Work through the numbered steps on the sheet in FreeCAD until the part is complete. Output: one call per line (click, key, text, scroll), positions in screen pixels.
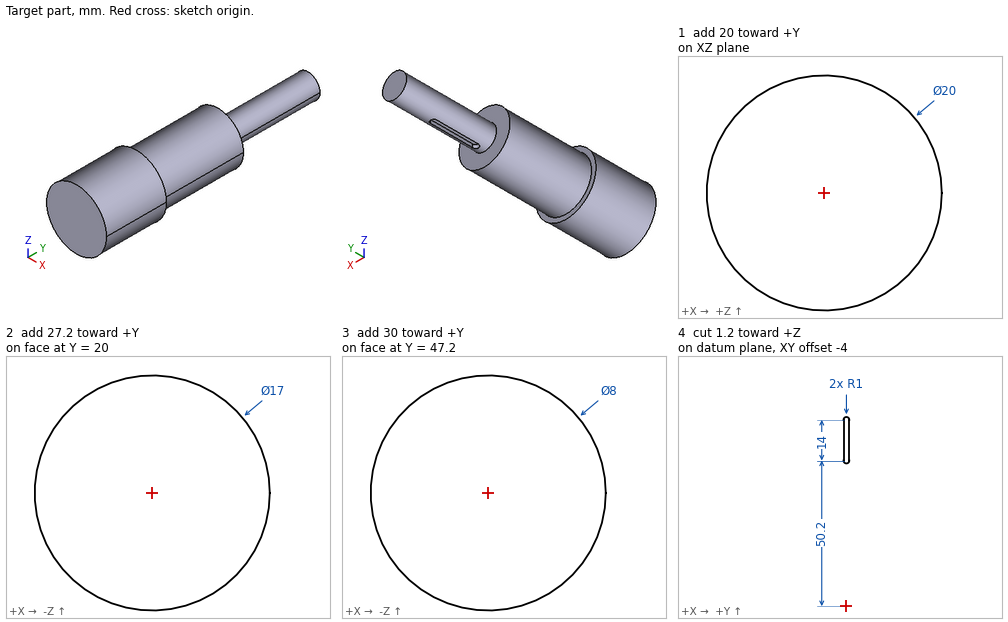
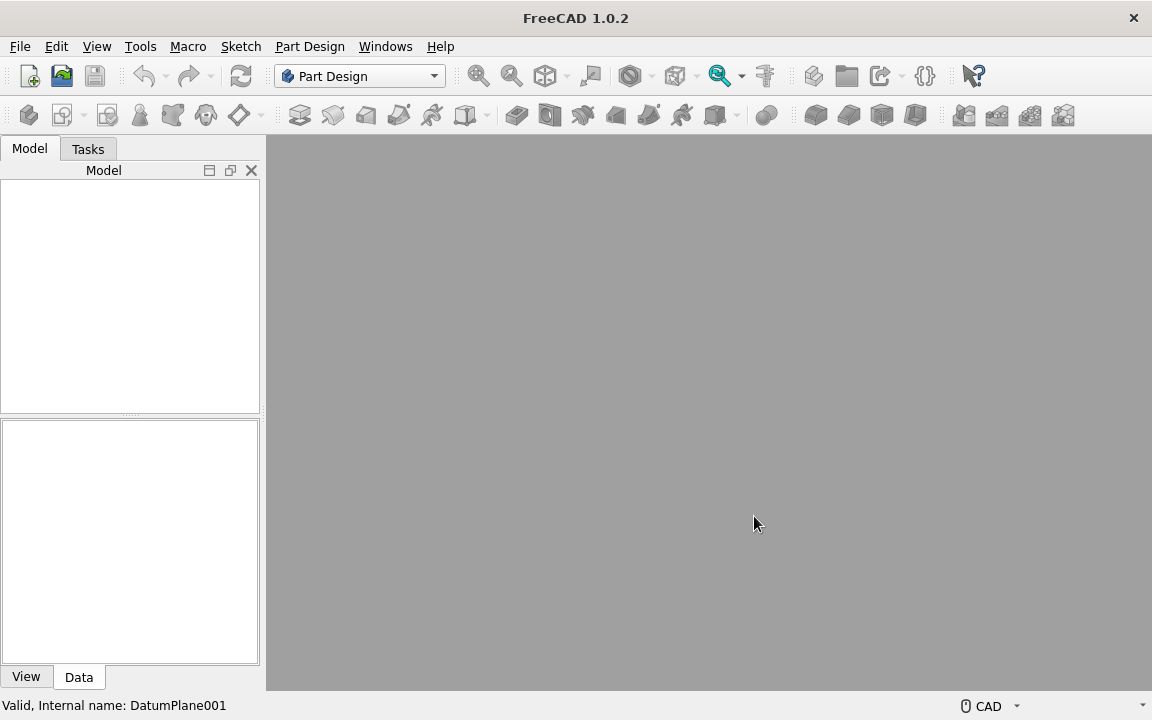
click(29, 76)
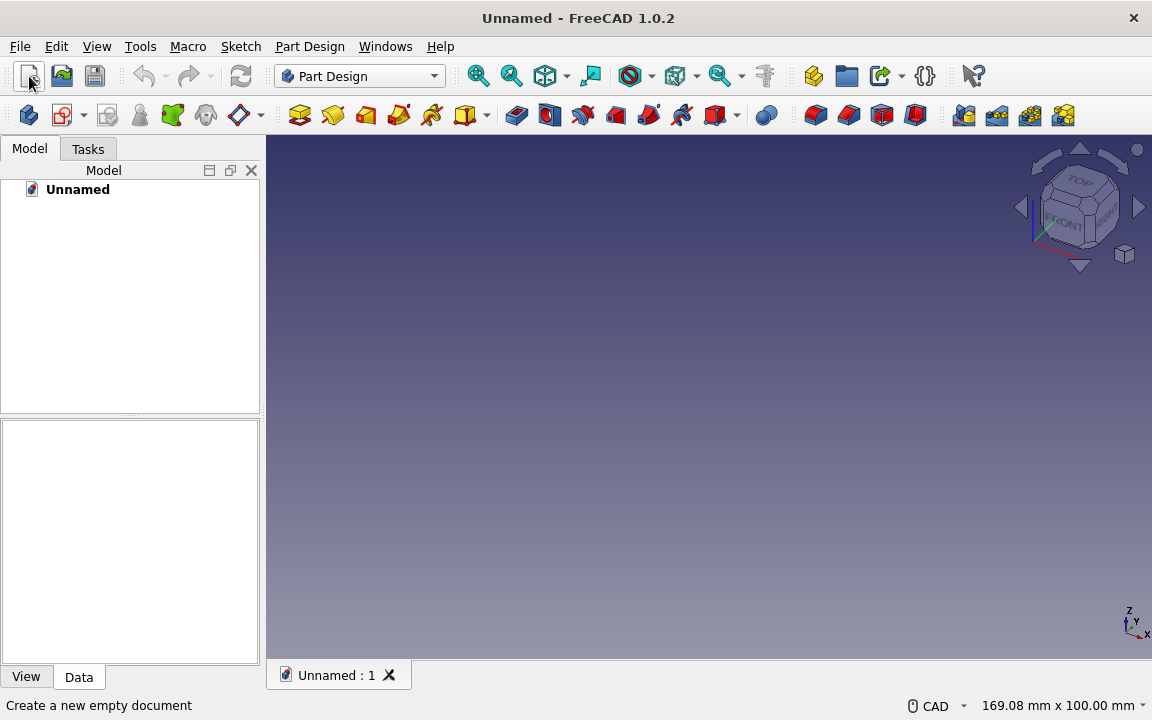
click(62, 116)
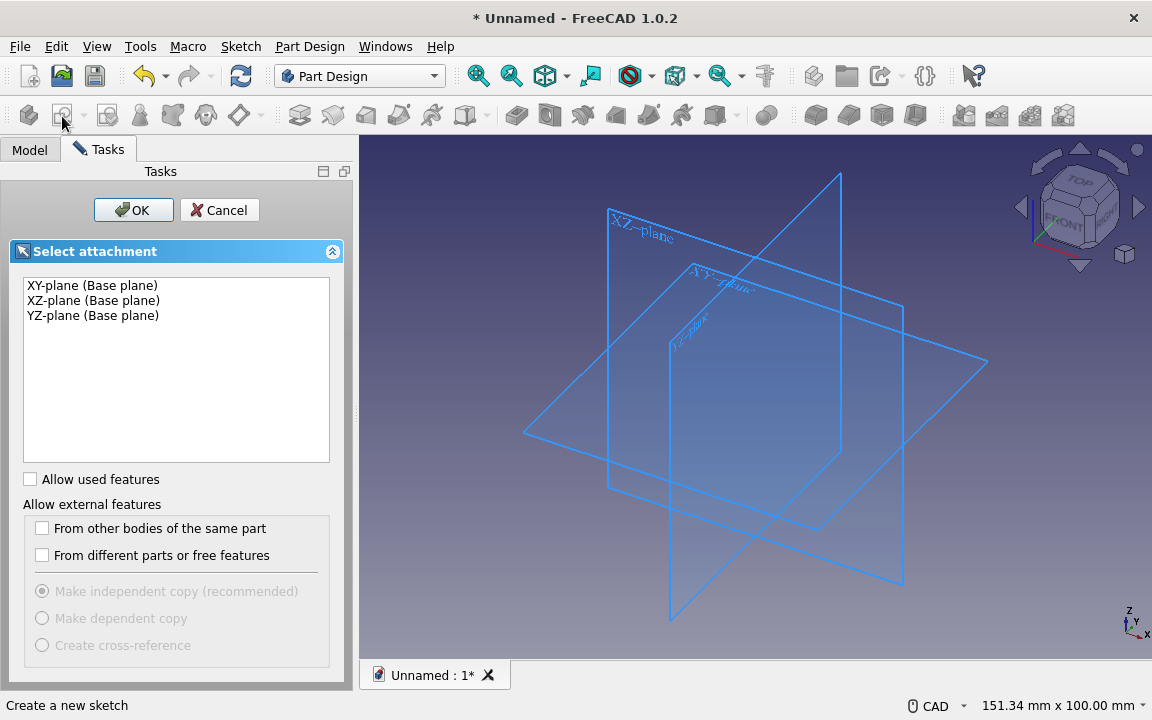
click(84, 300)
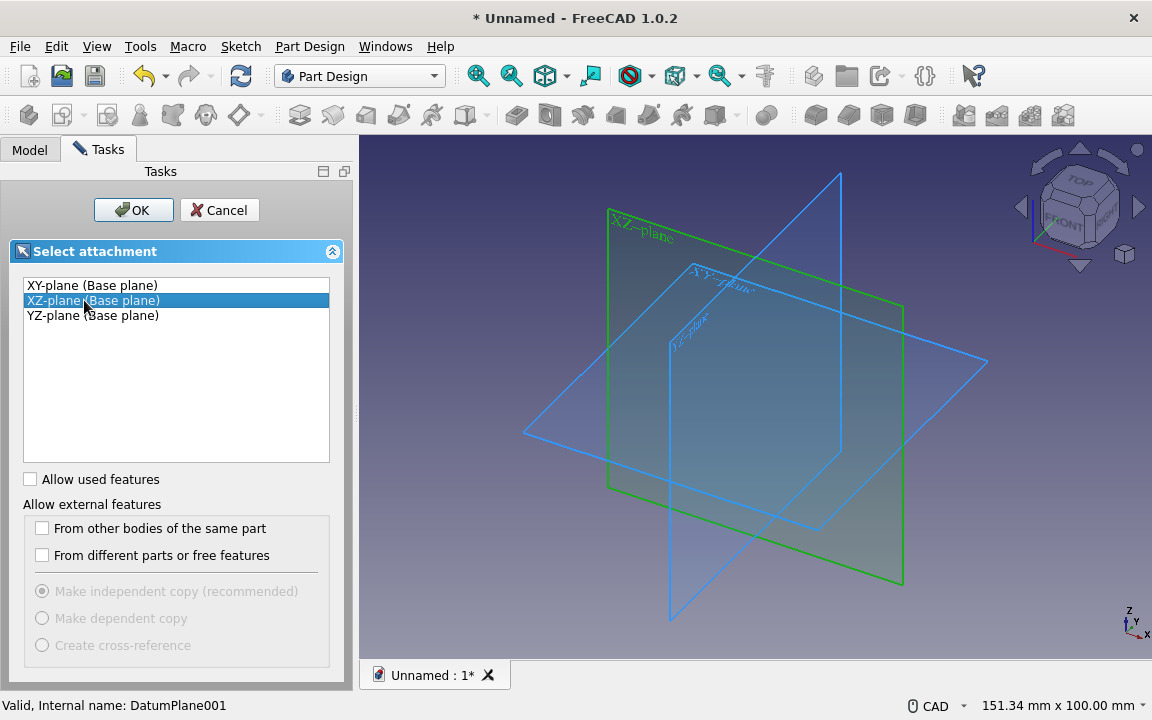
click(134, 210)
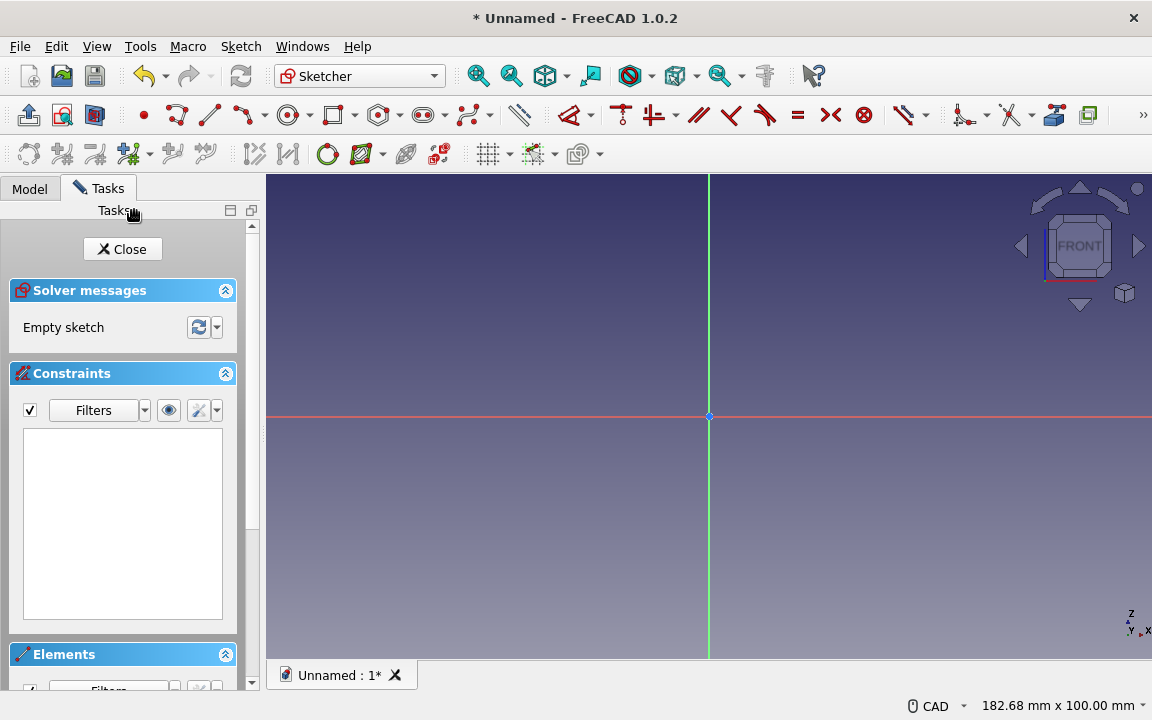
scroll(739, 416, up, 6)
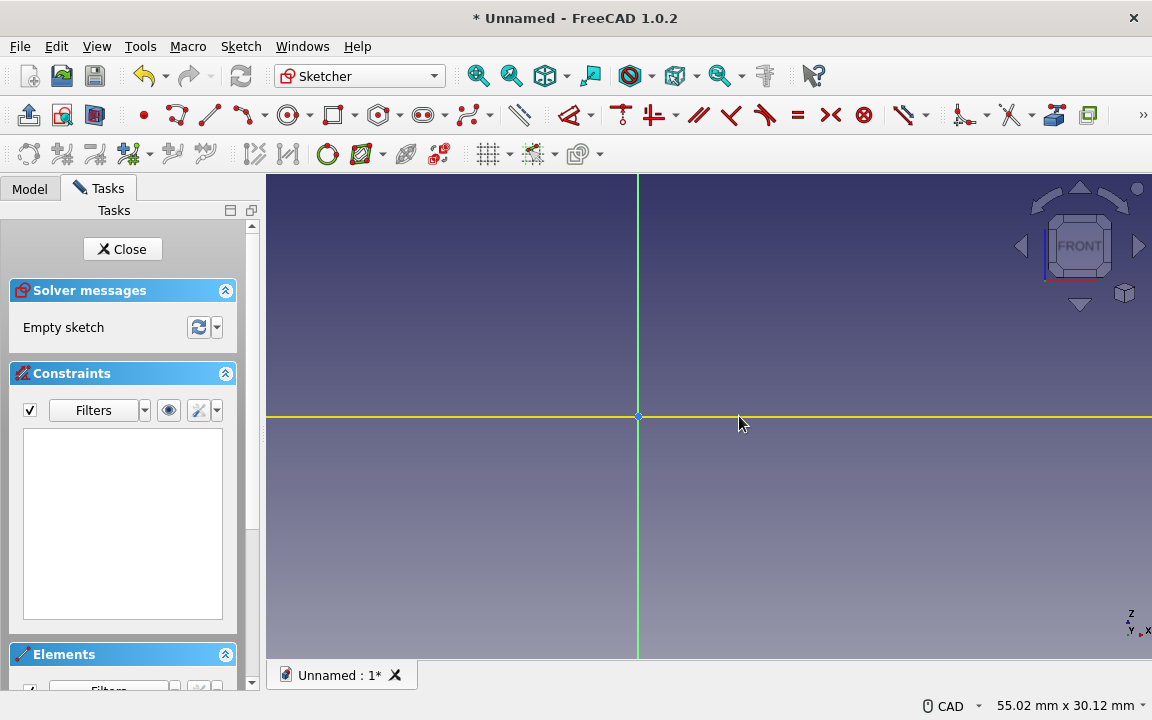
click(288, 116)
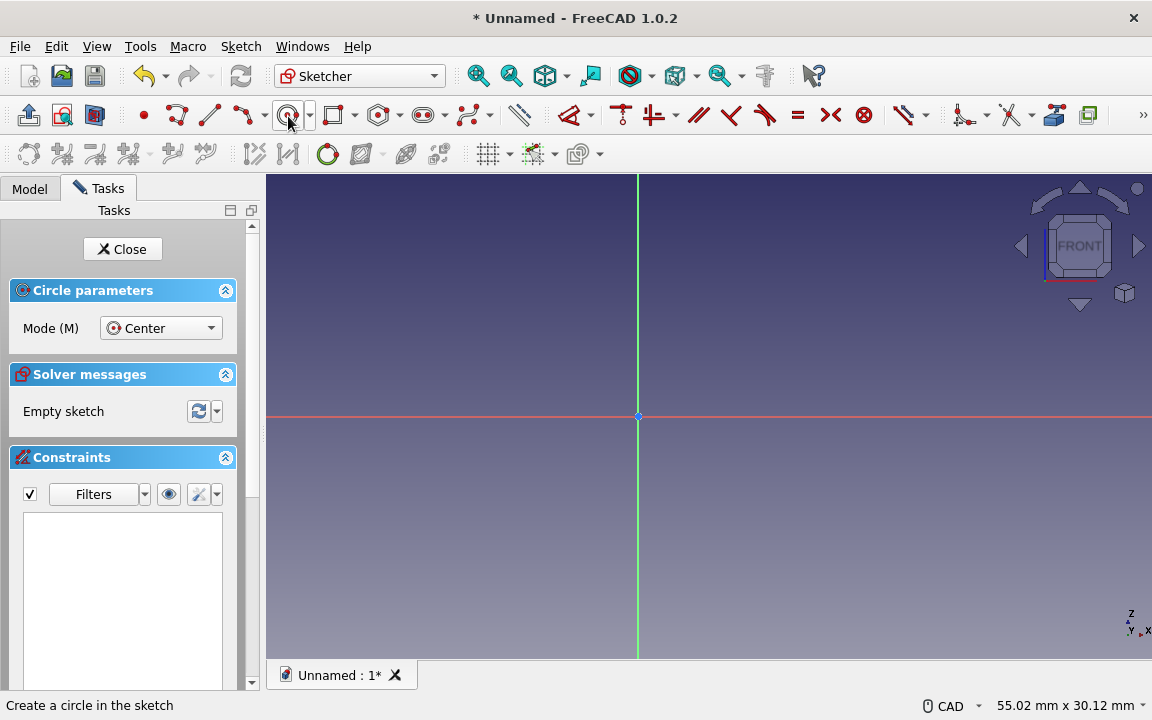
click(638, 416)
move(752, 303)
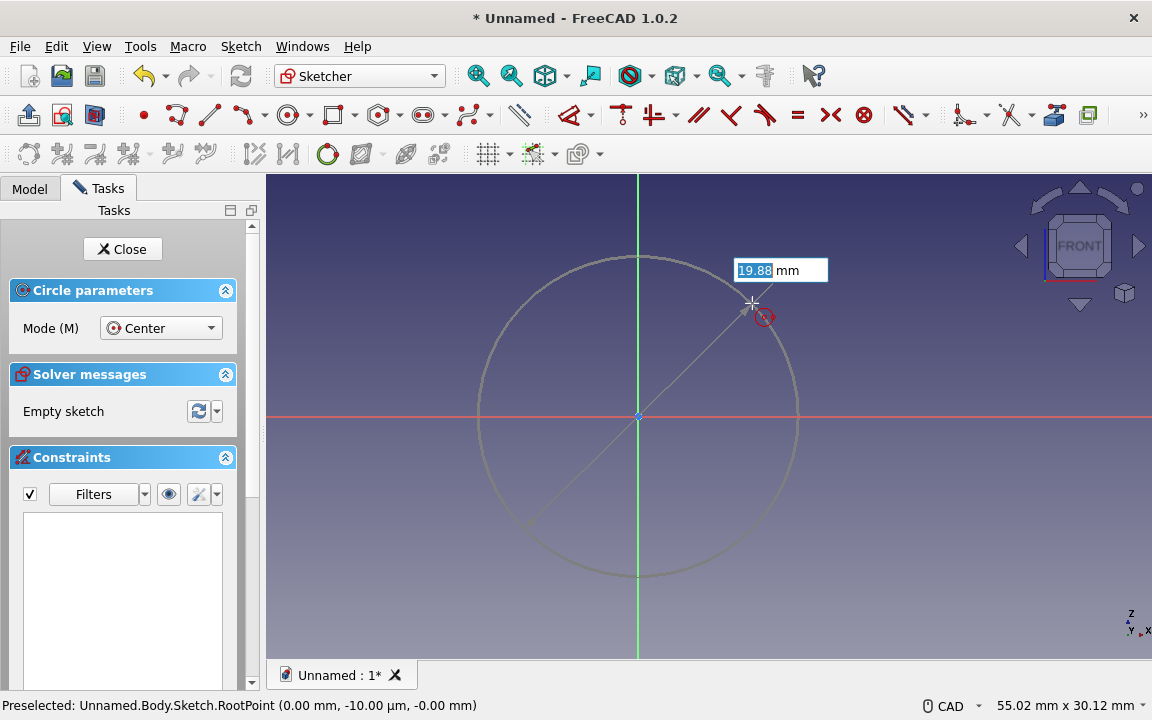
text(20)
key(Return)
key(Escape)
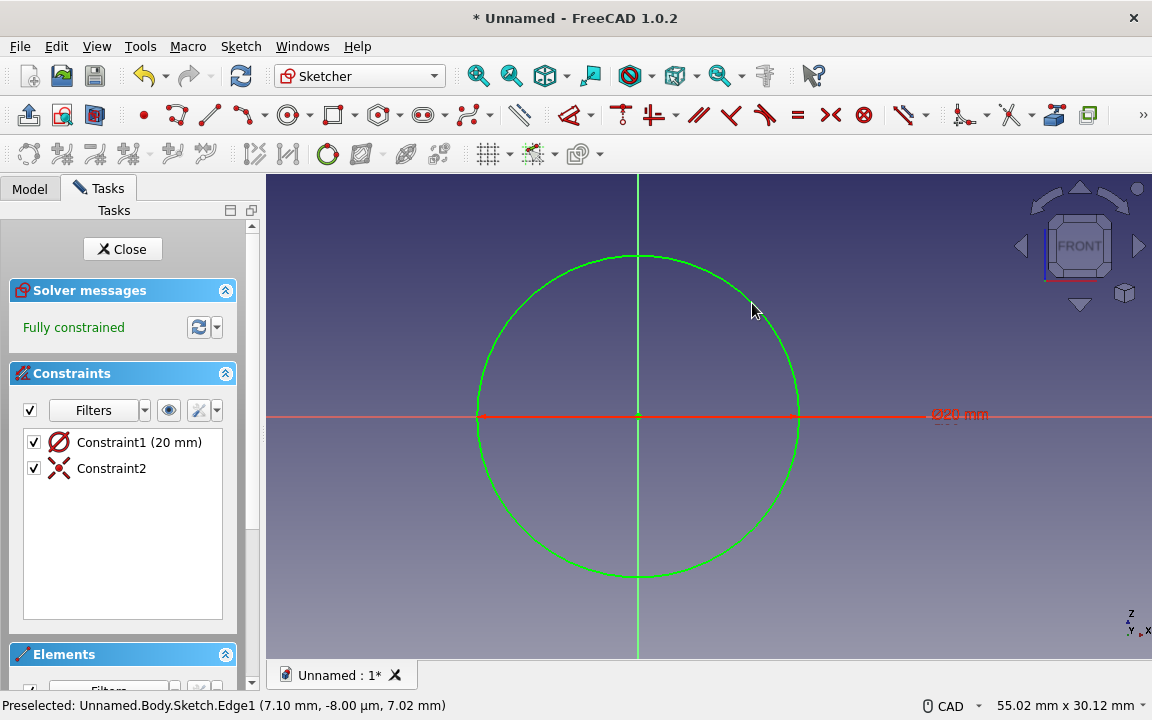
click(123, 249)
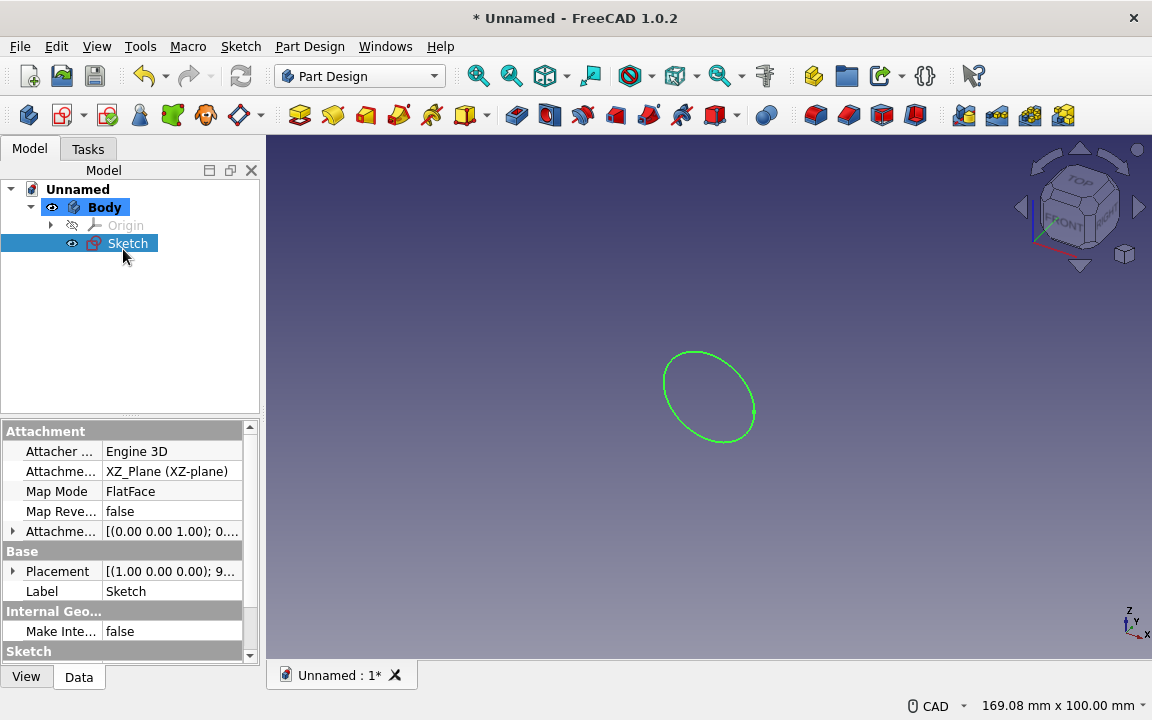
click(300, 116)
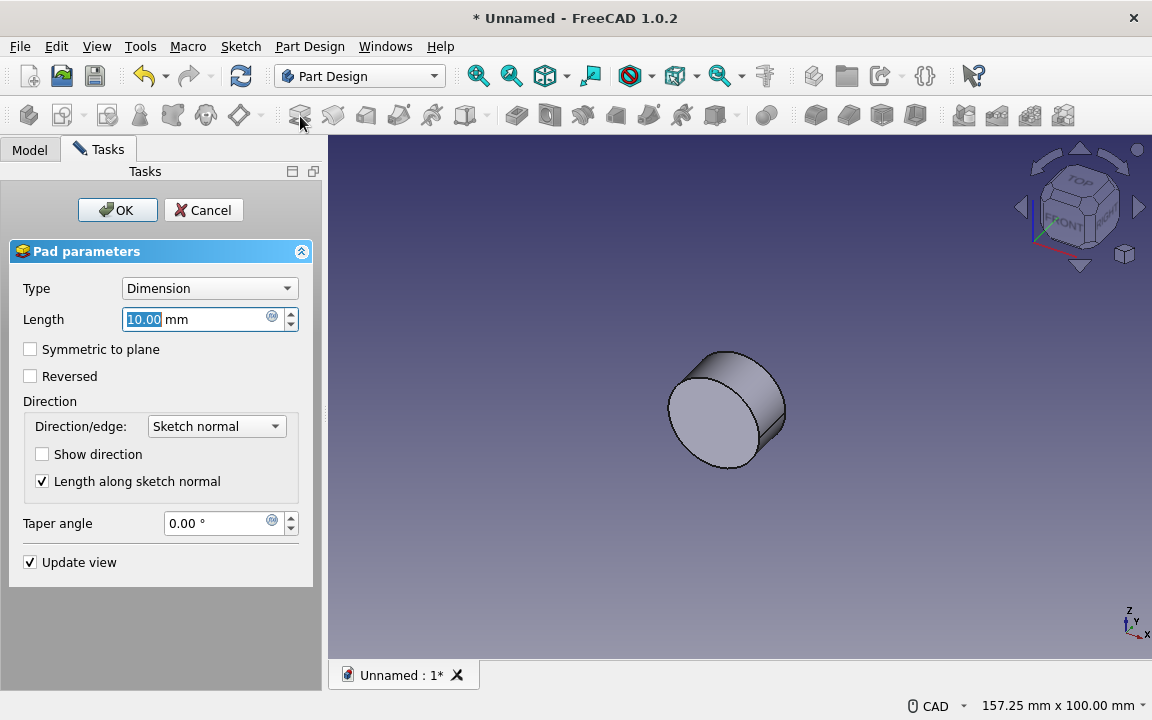
text(20)
key(Tab)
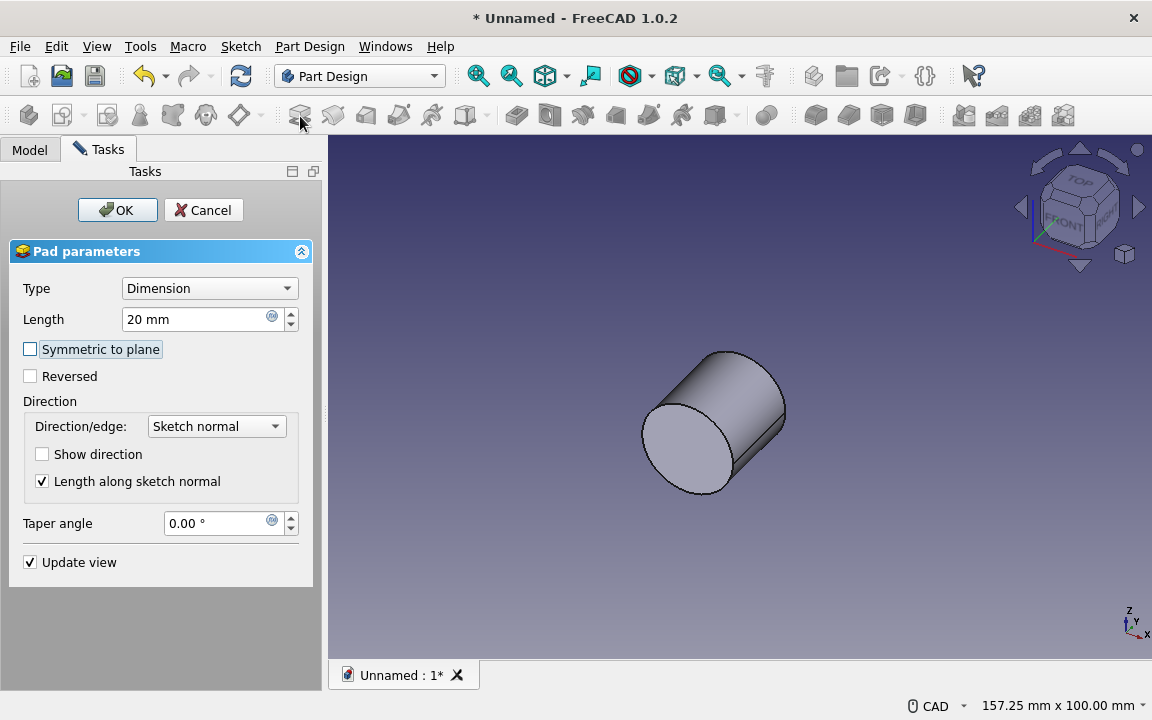
click(31, 376)